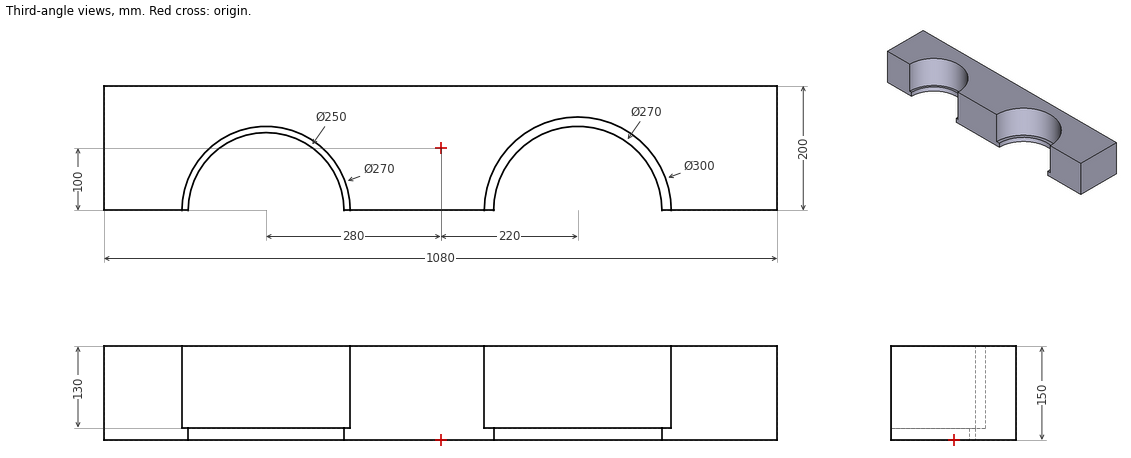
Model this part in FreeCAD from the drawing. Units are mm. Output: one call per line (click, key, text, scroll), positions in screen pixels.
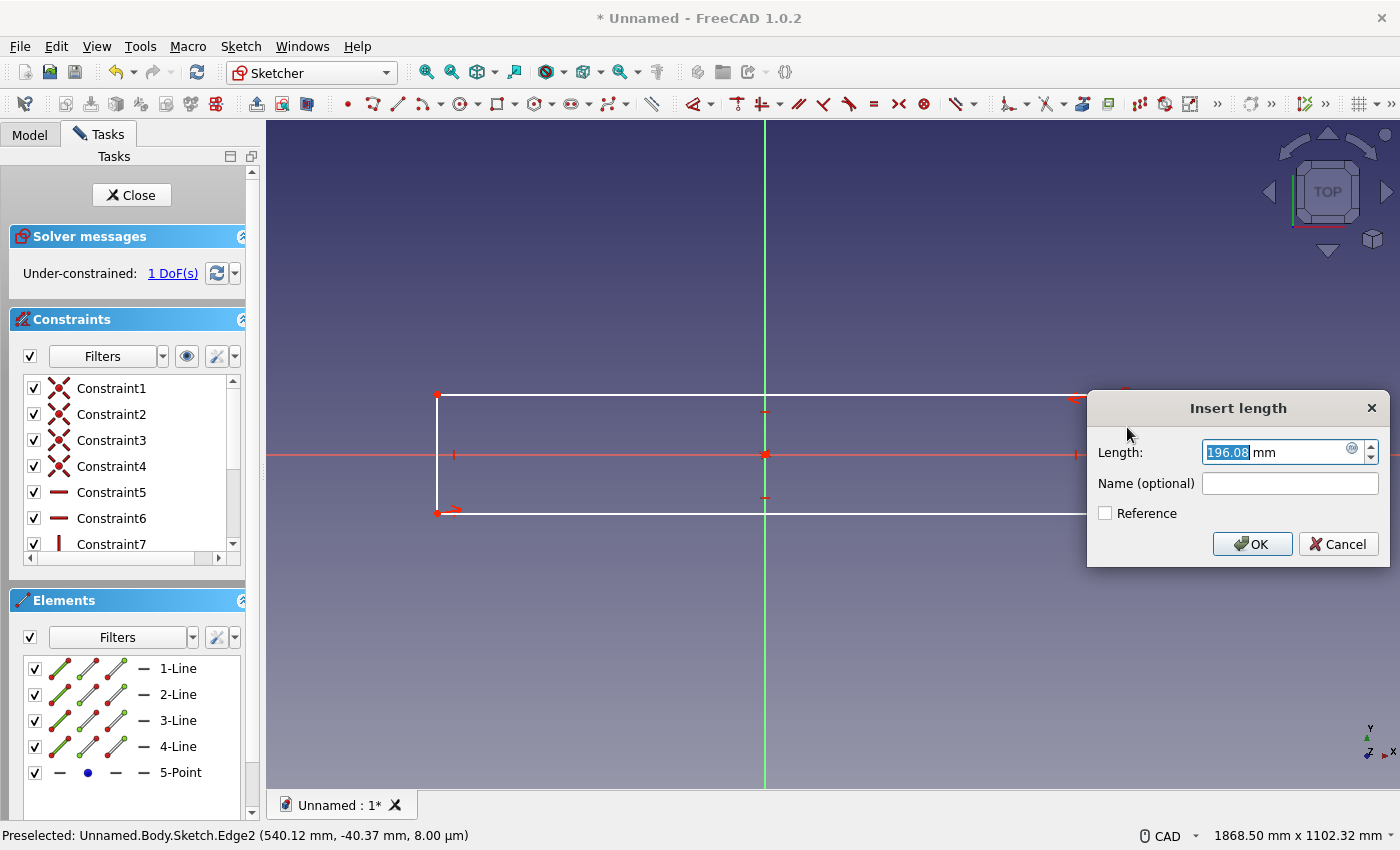
text(200)
key(Return)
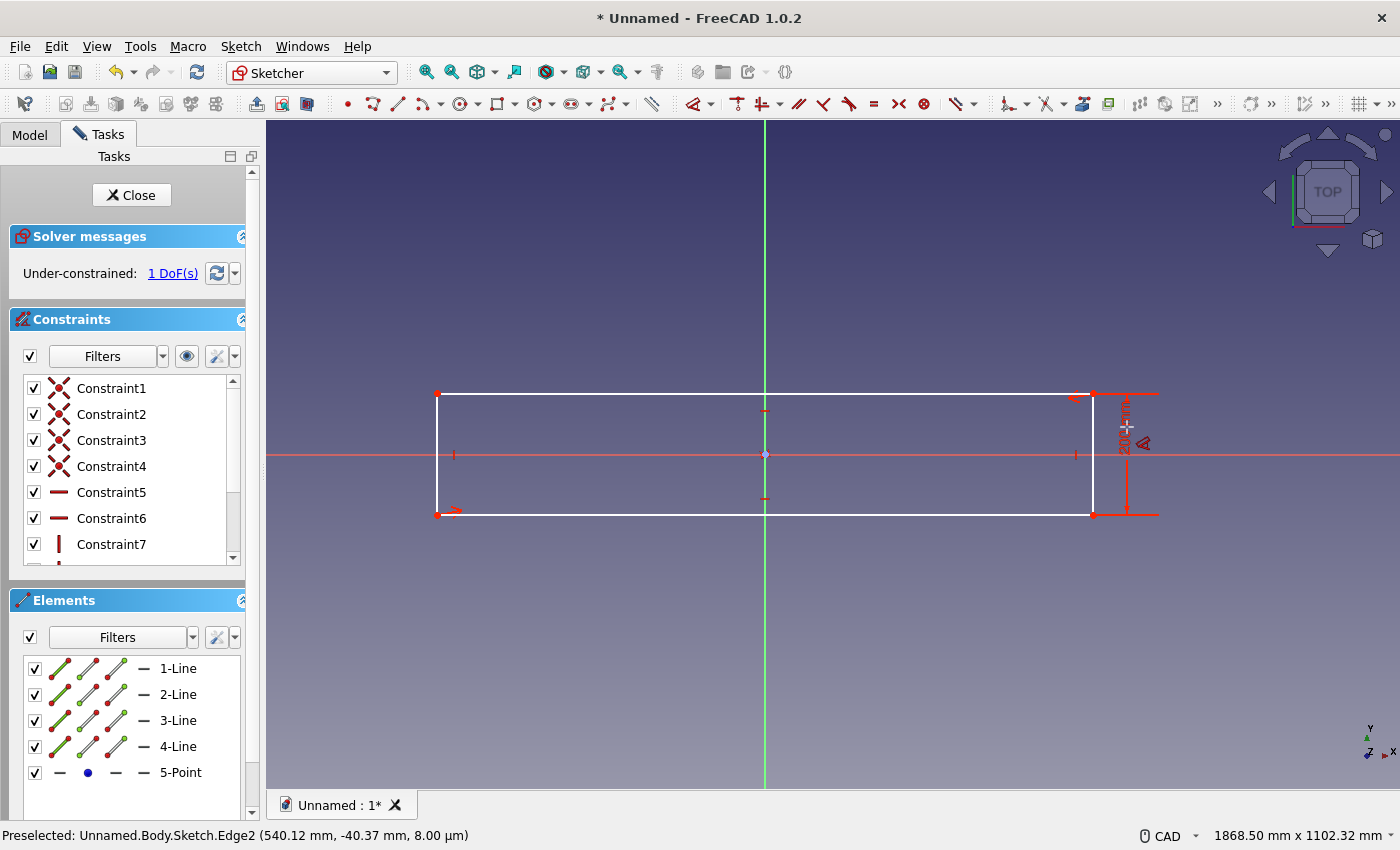
click(634, 515)
click(614, 549)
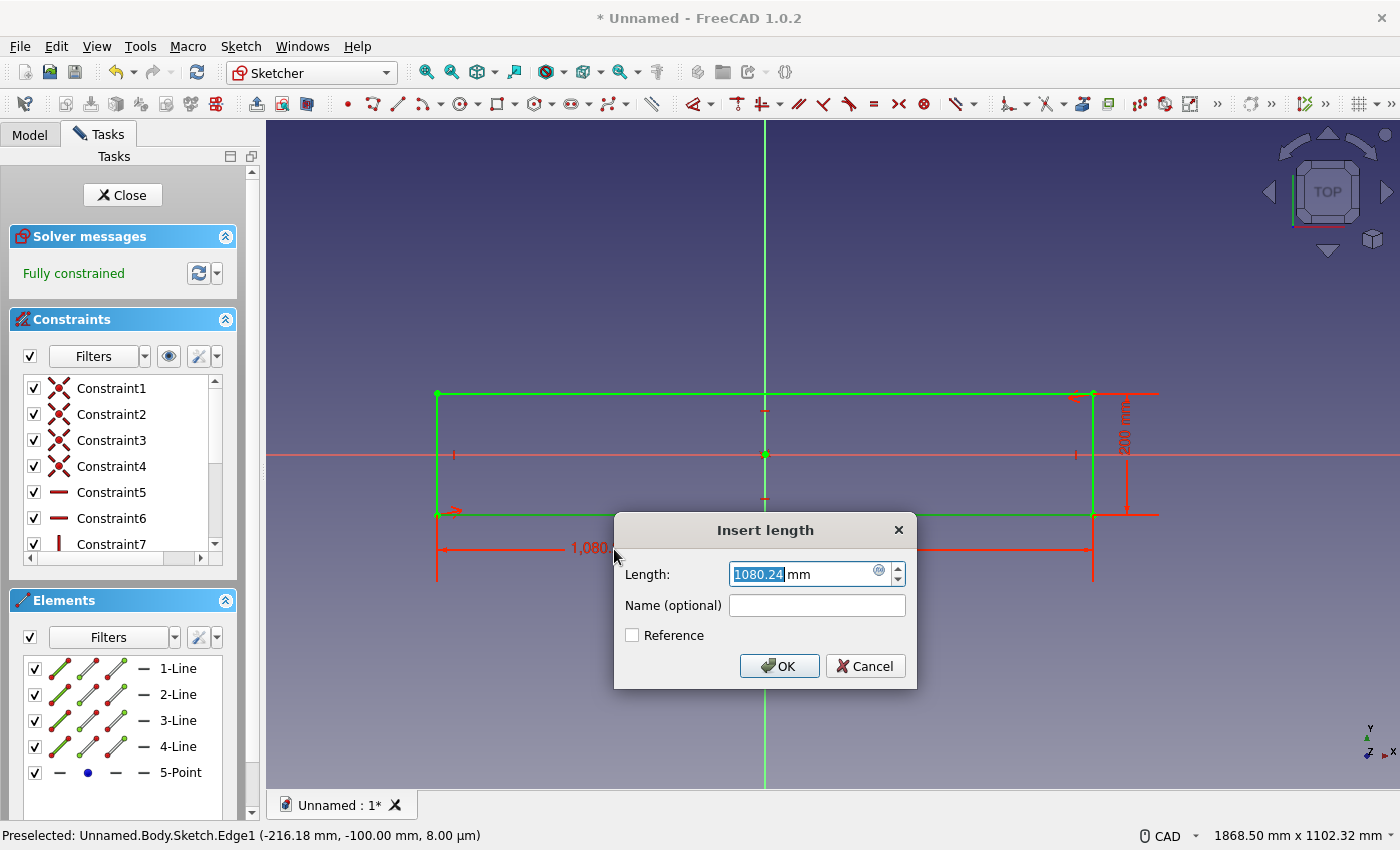
text(1080)
key(Return)
key(Escape)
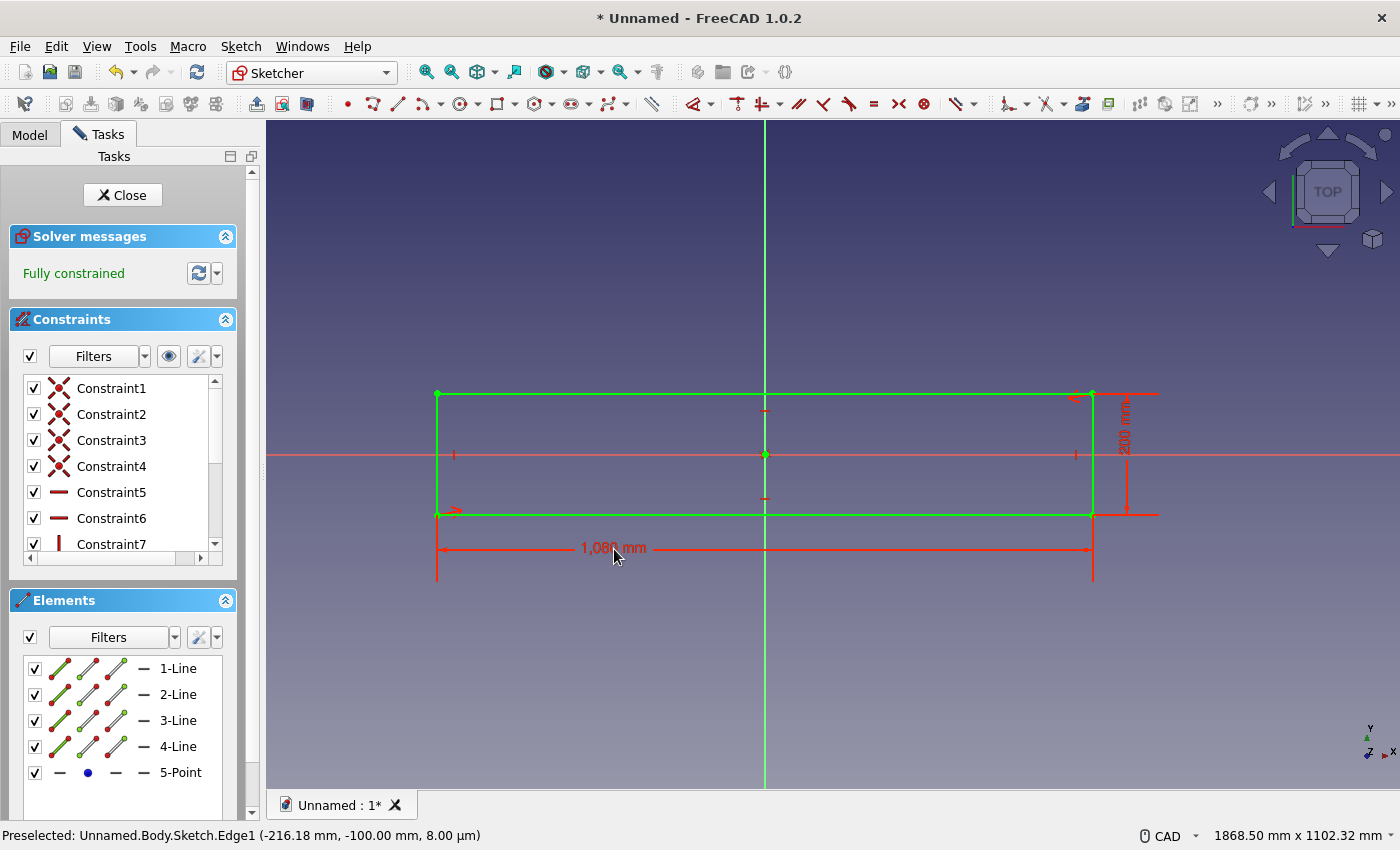
click(123, 195)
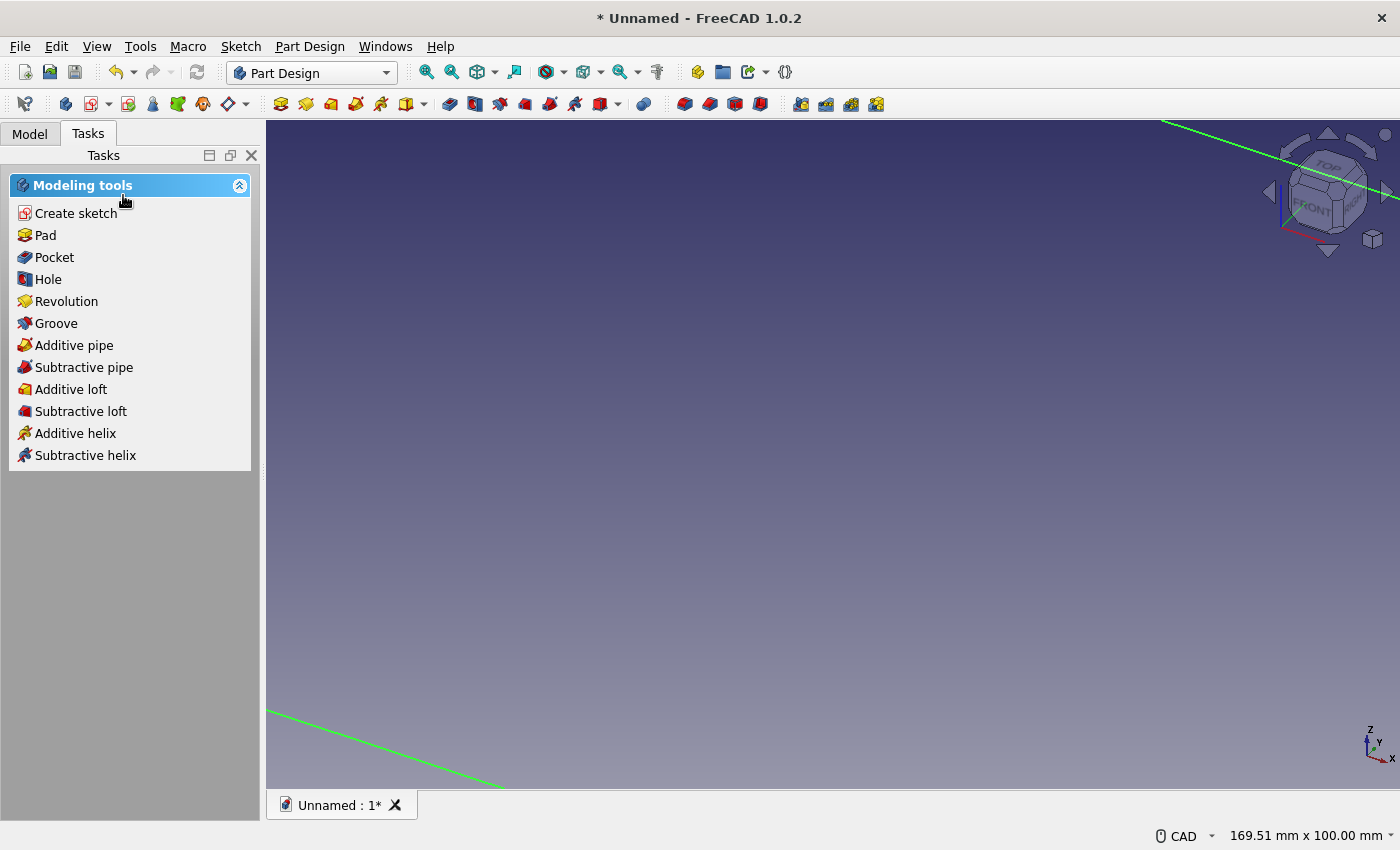
click(281, 104)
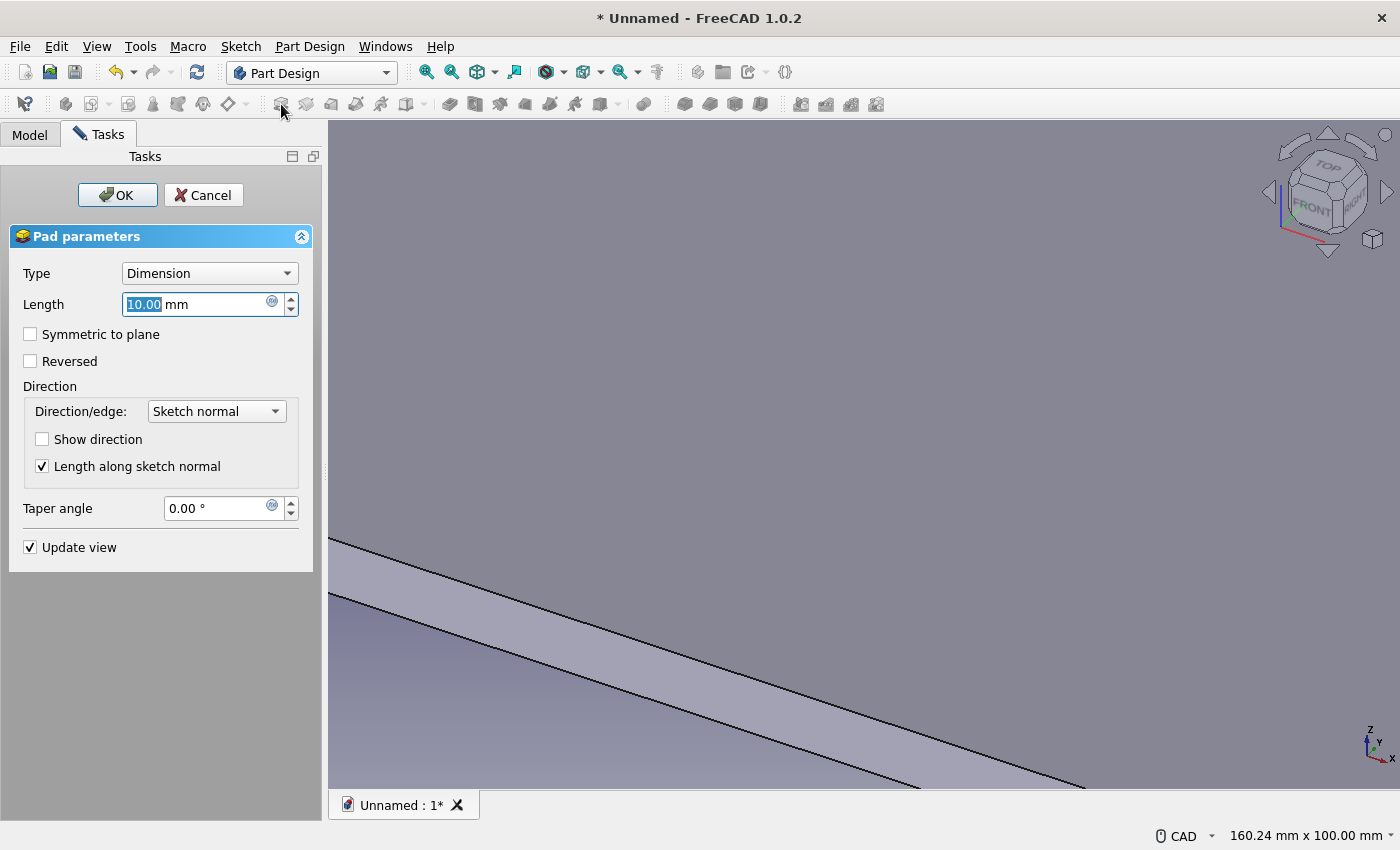
text(150)
key(Tab)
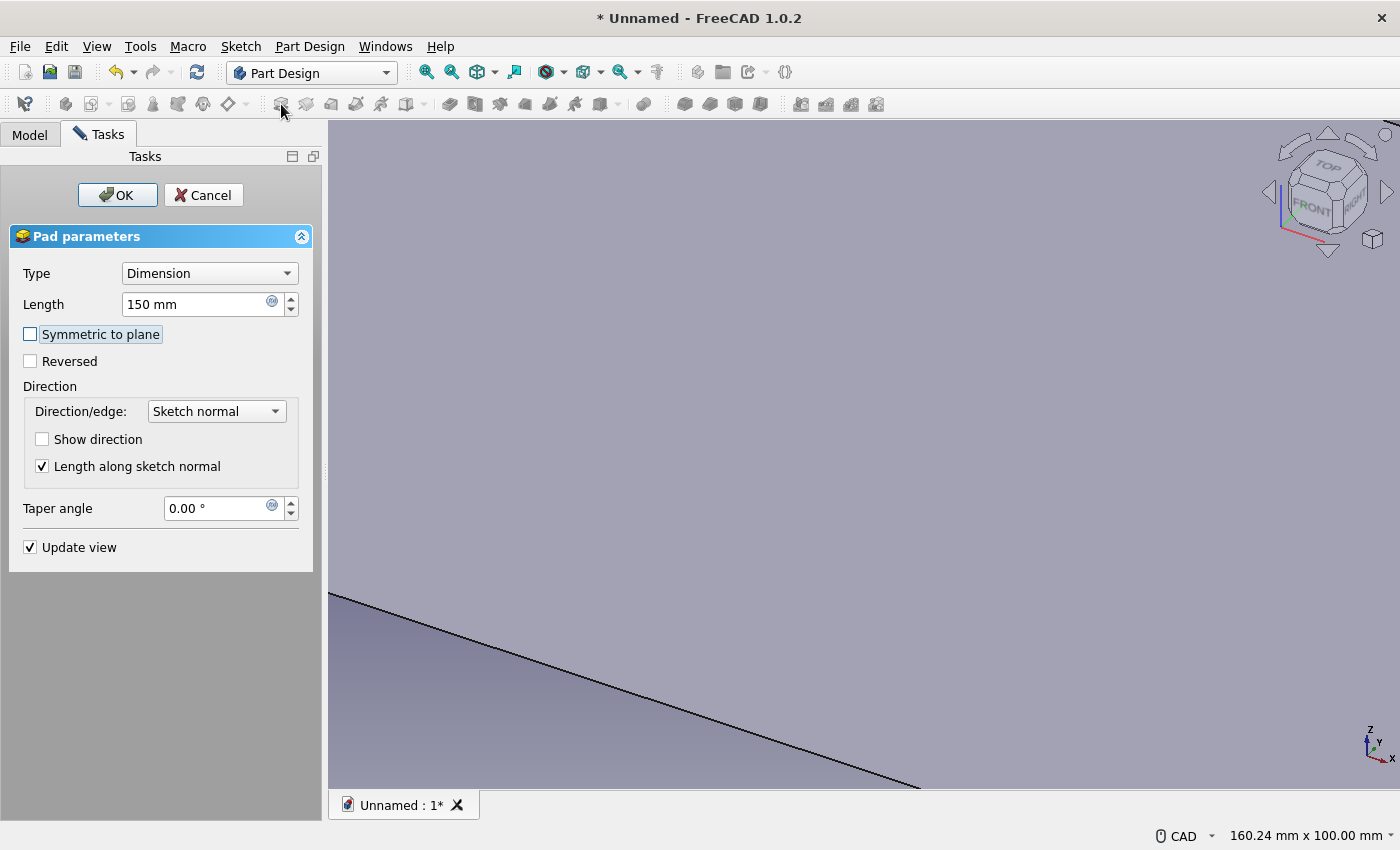
click(118, 195)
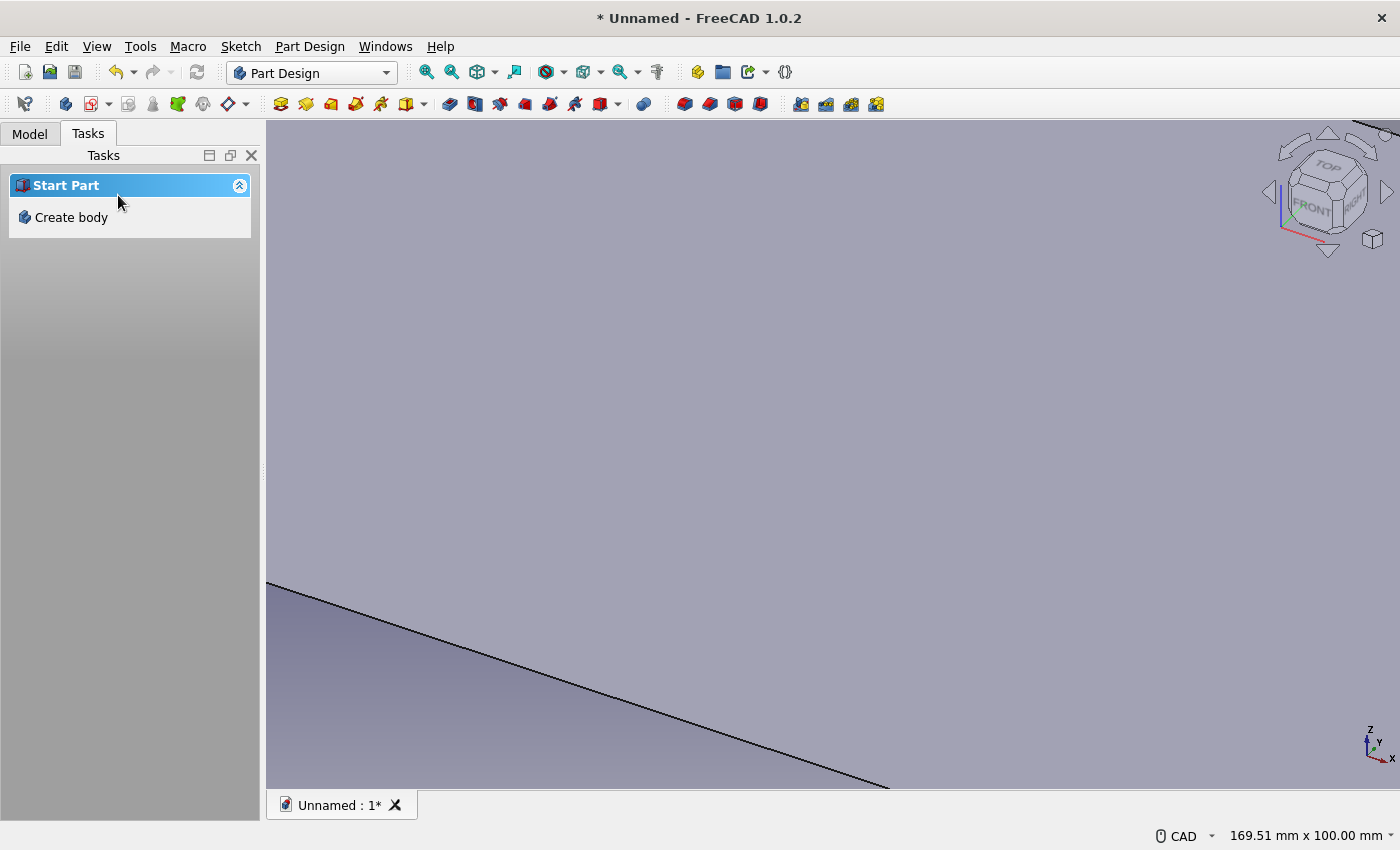
key(v)
key(f)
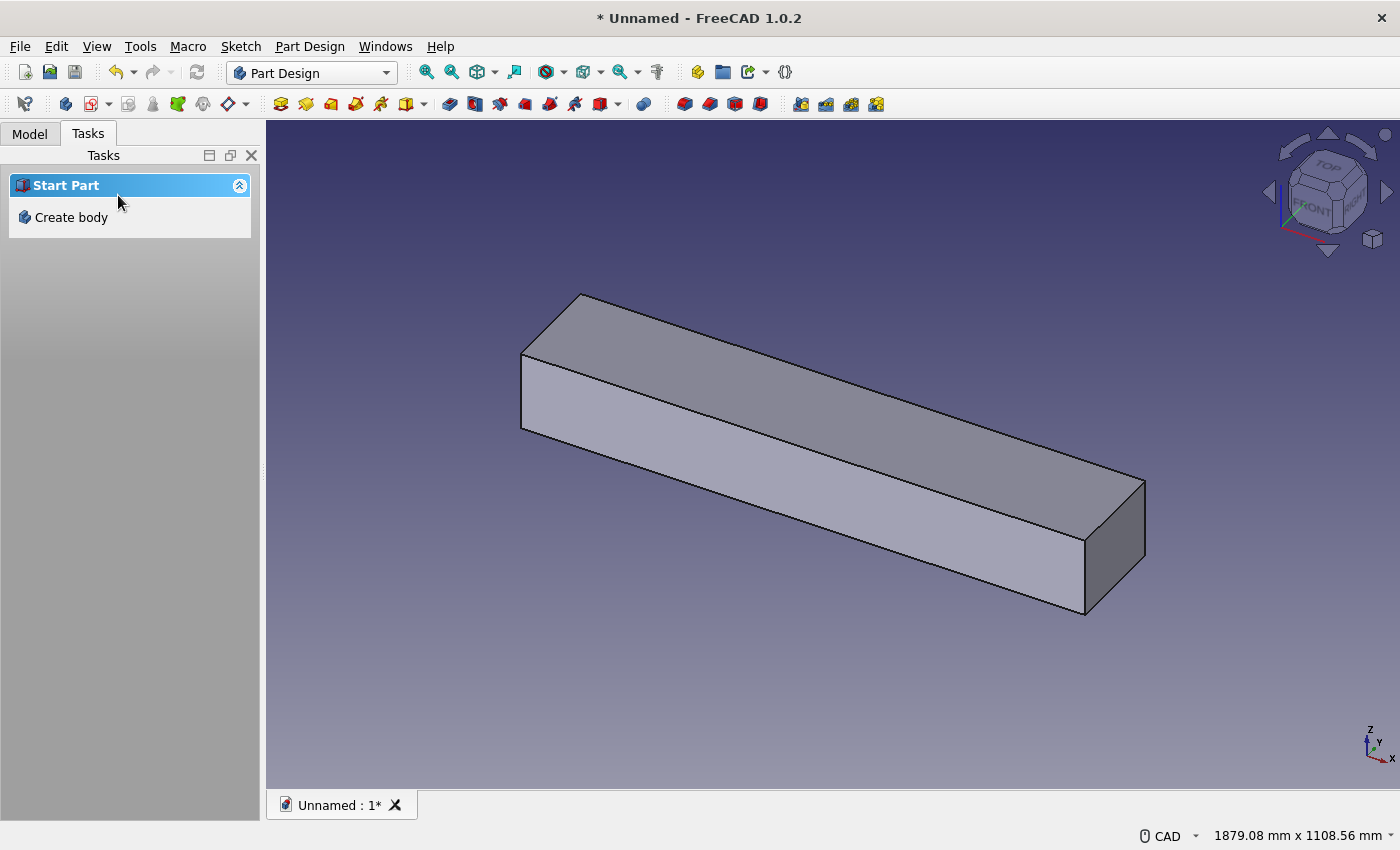
click(994, 470)